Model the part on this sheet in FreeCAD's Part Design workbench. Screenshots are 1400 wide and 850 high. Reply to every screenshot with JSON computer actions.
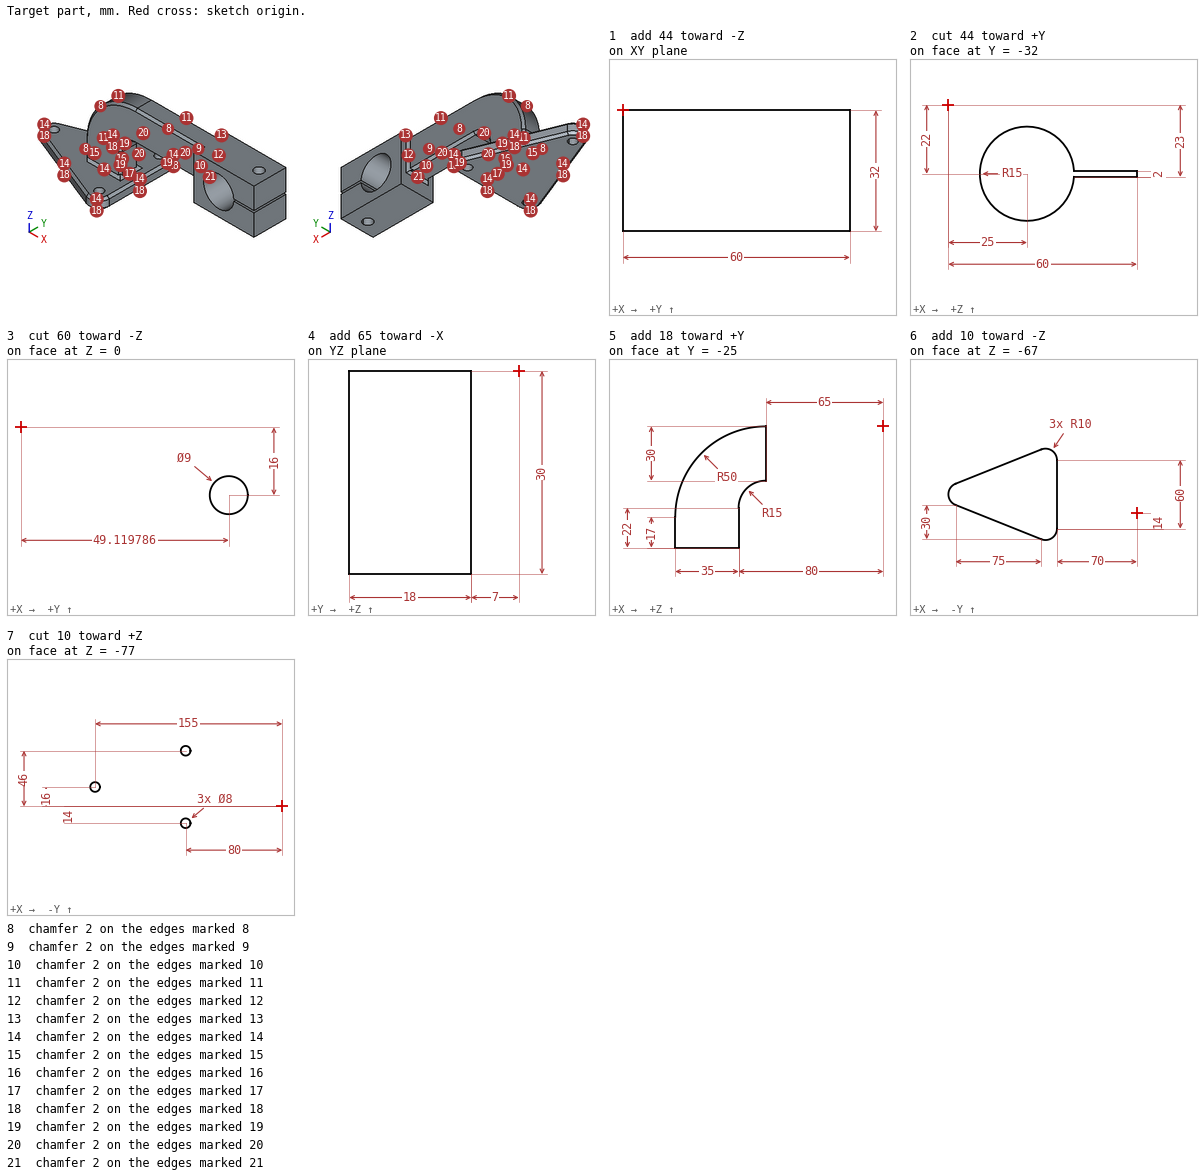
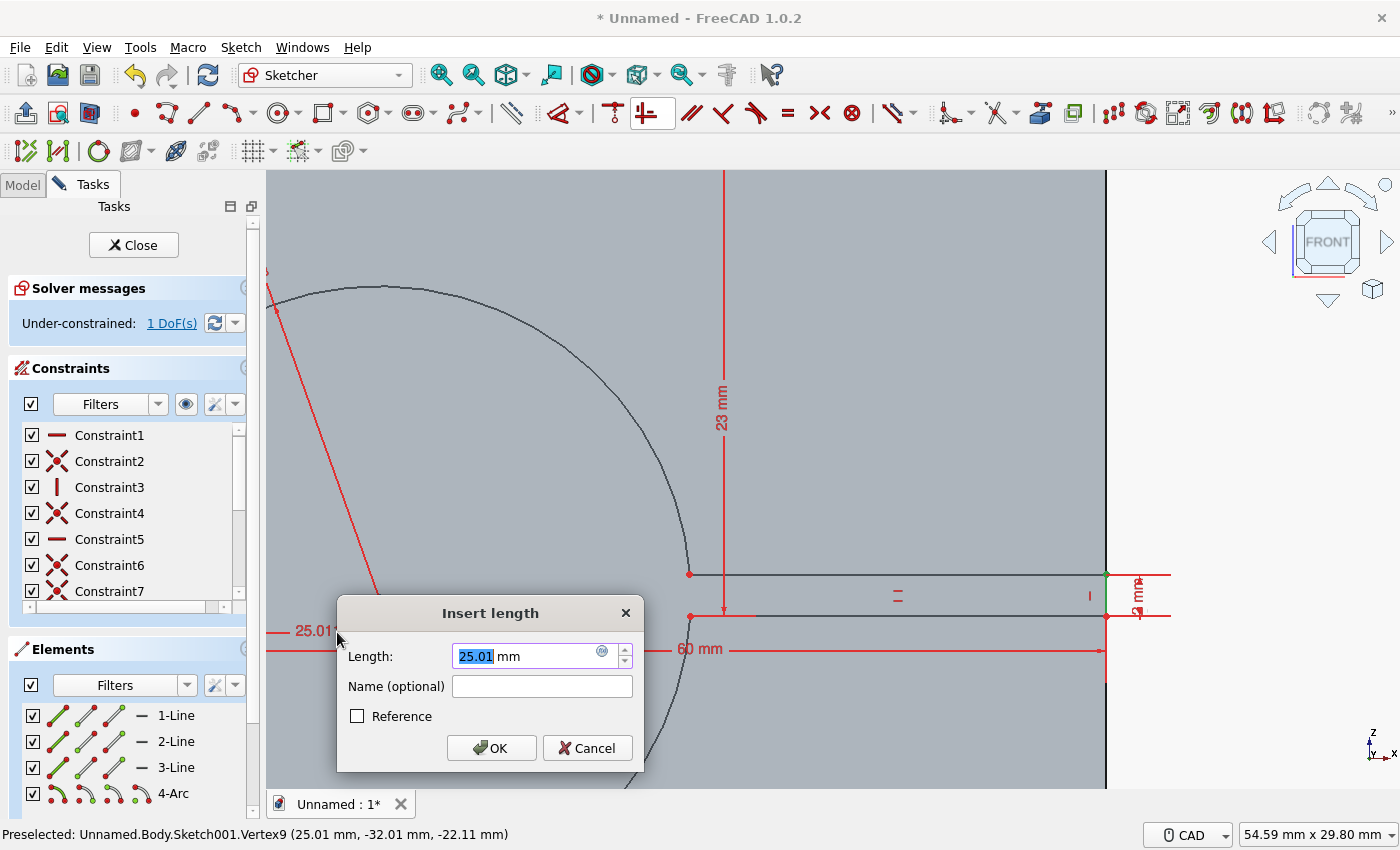
{"action": "type", "text": "25"}
{"action": "key", "text": "Return"}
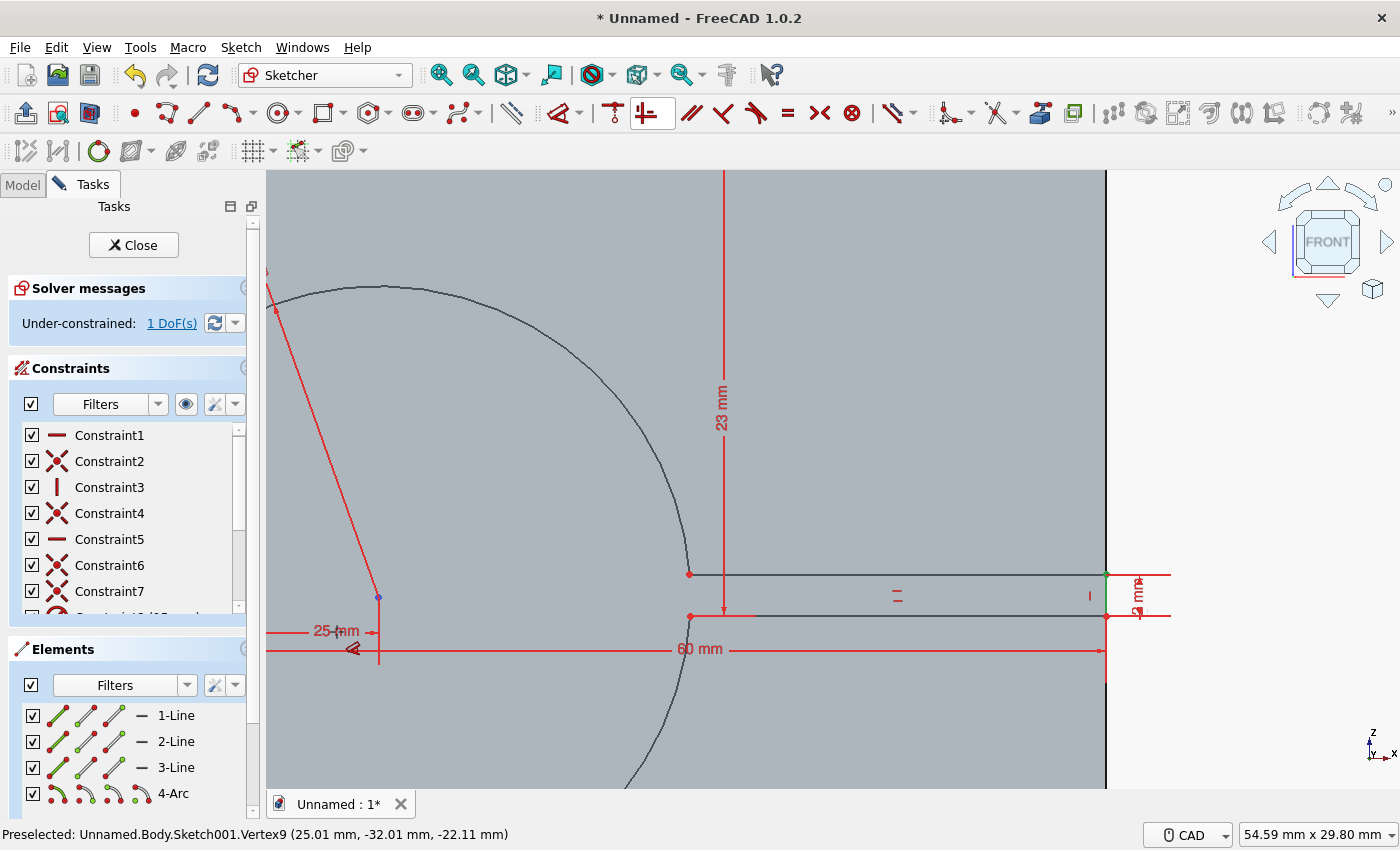
{"action": "left_click", "coordinate": [379, 598]}
{"action": "left_click", "coordinate": [413, 398]}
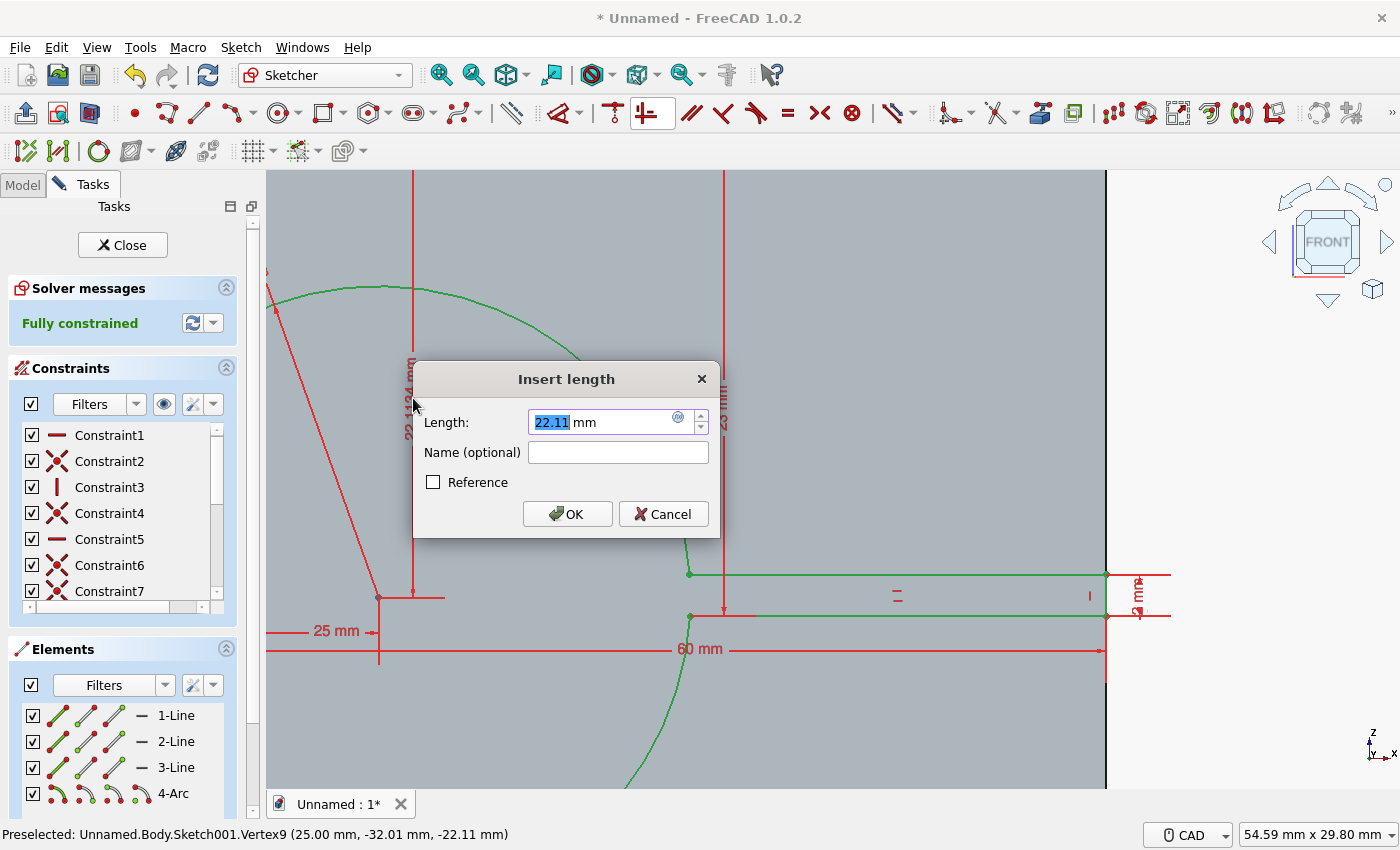
{"action": "type", "text": "22"}
{"action": "key", "text": "Return"}
{"action": "key", "text": "Escape"}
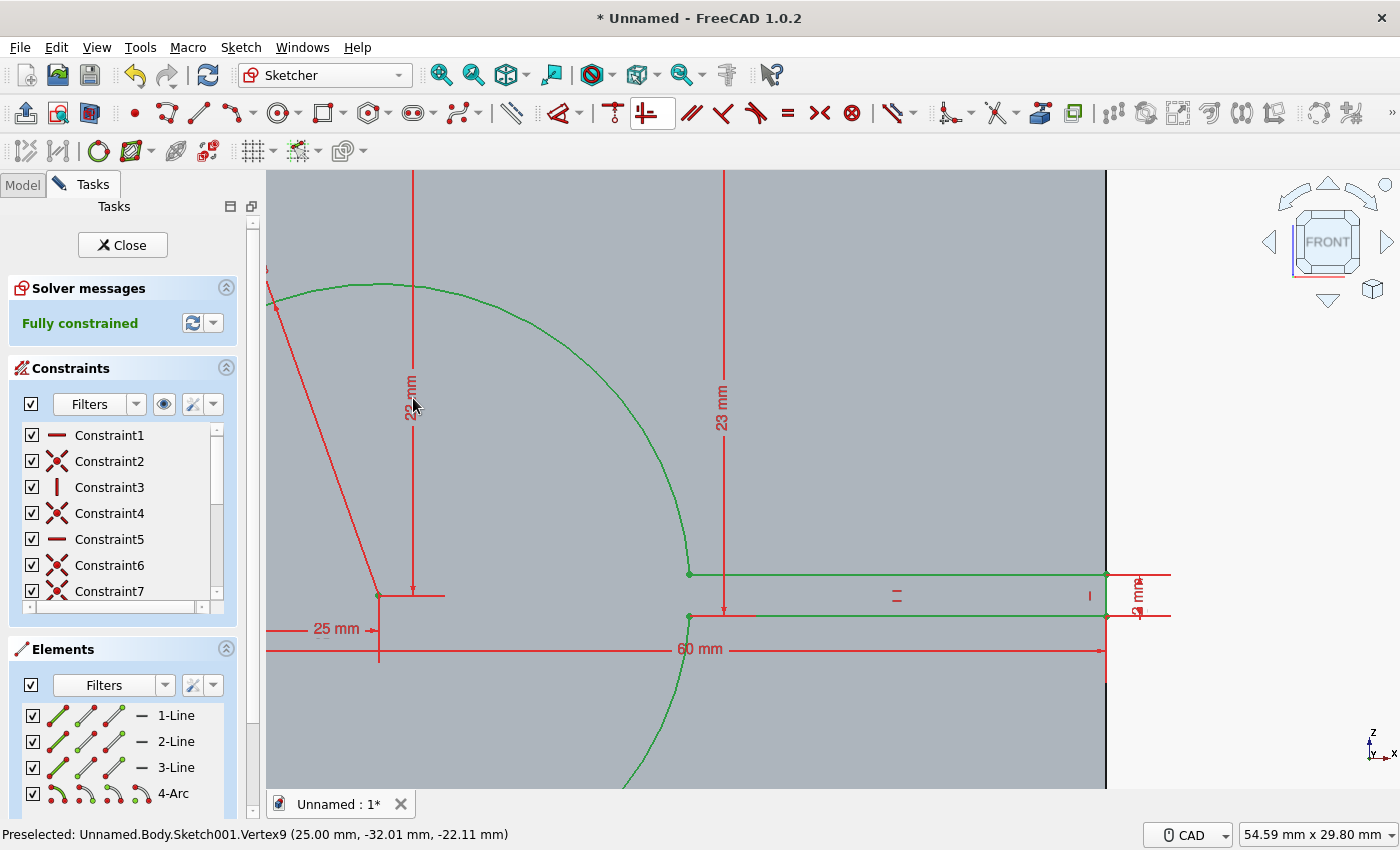
{"action": "left_click", "coordinate": [123, 245]}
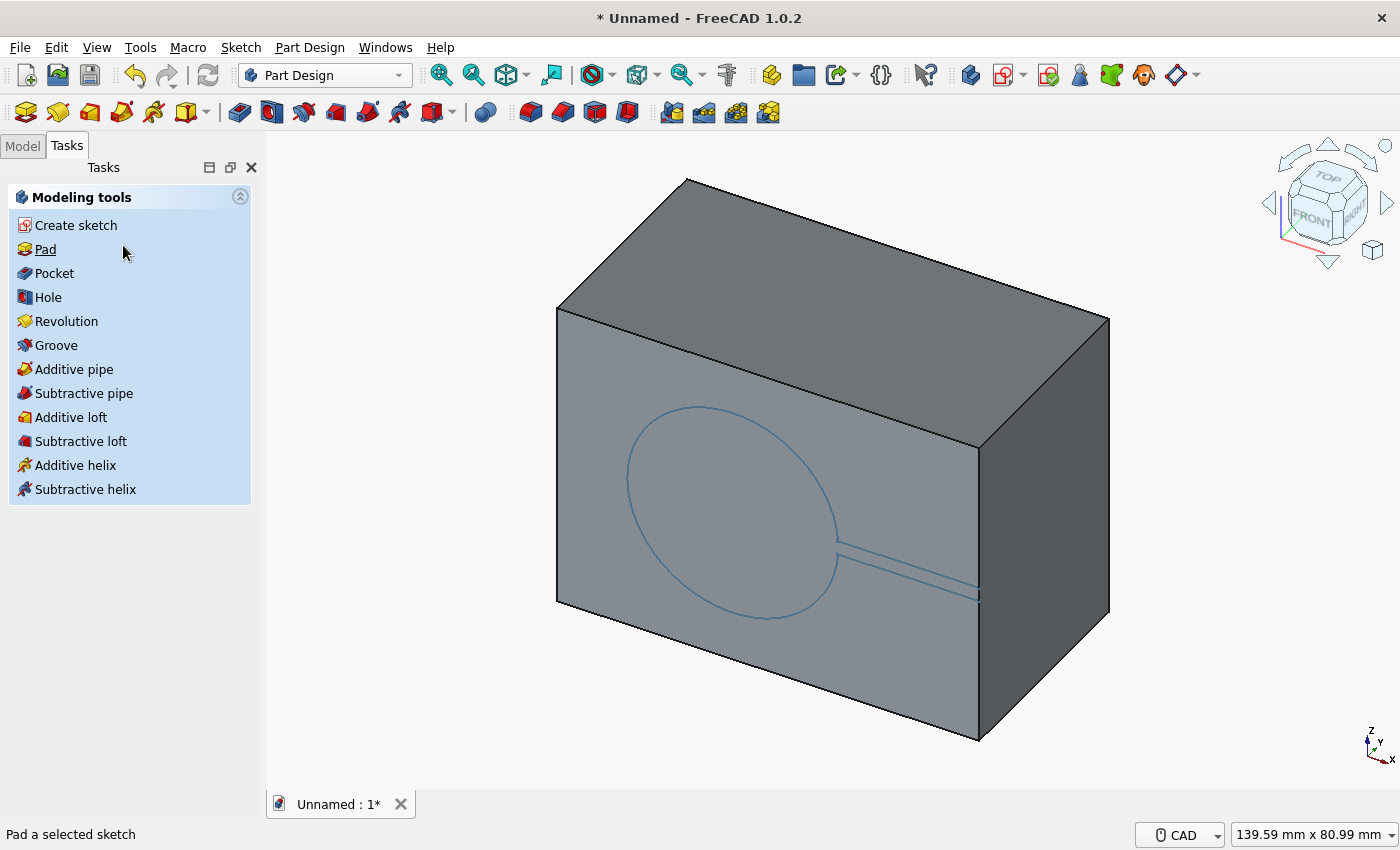
{"action": "left_click", "coordinate": [240, 112]}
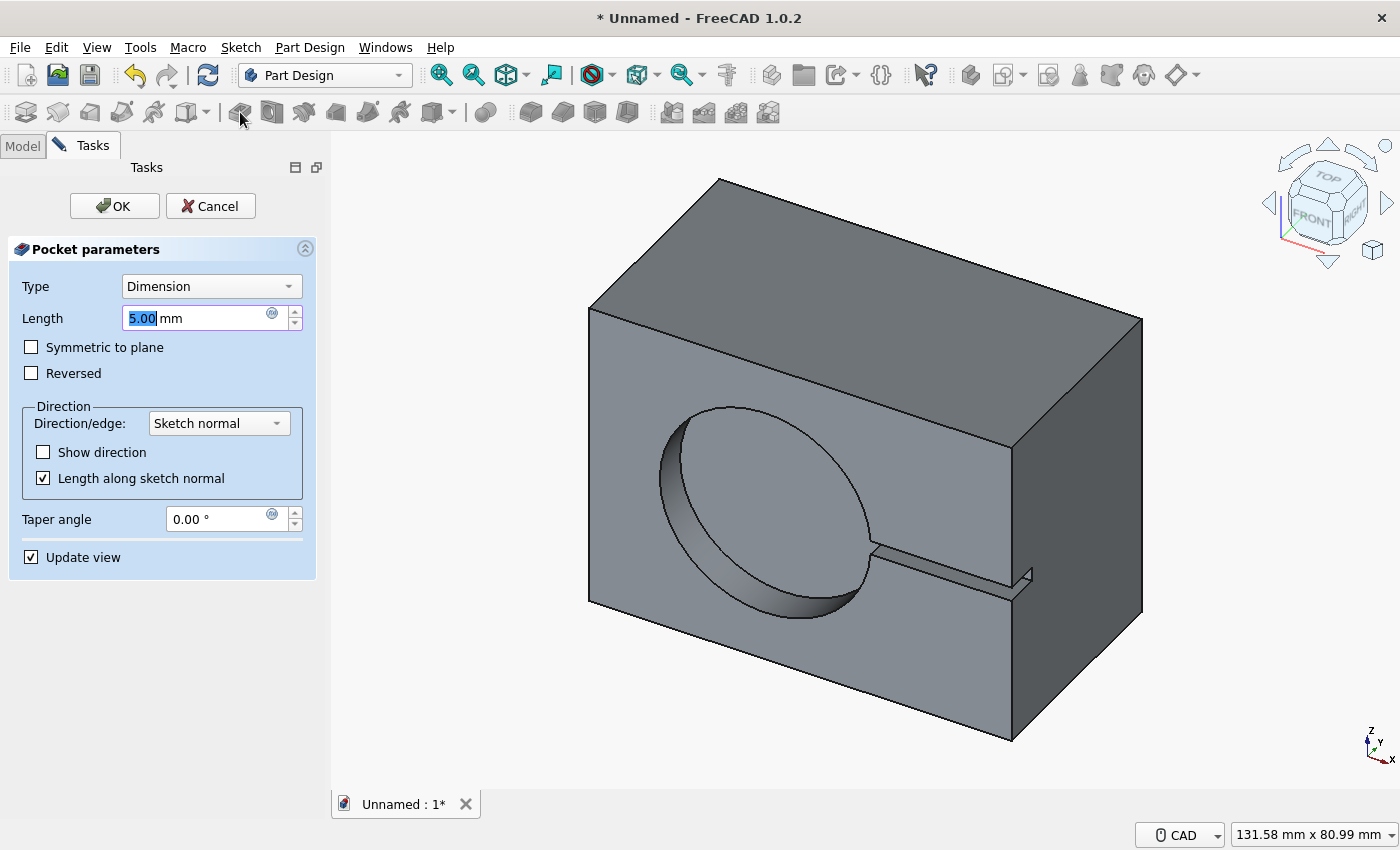
{"action": "type", "text": "44"}
{"action": "key", "text": "Tab"}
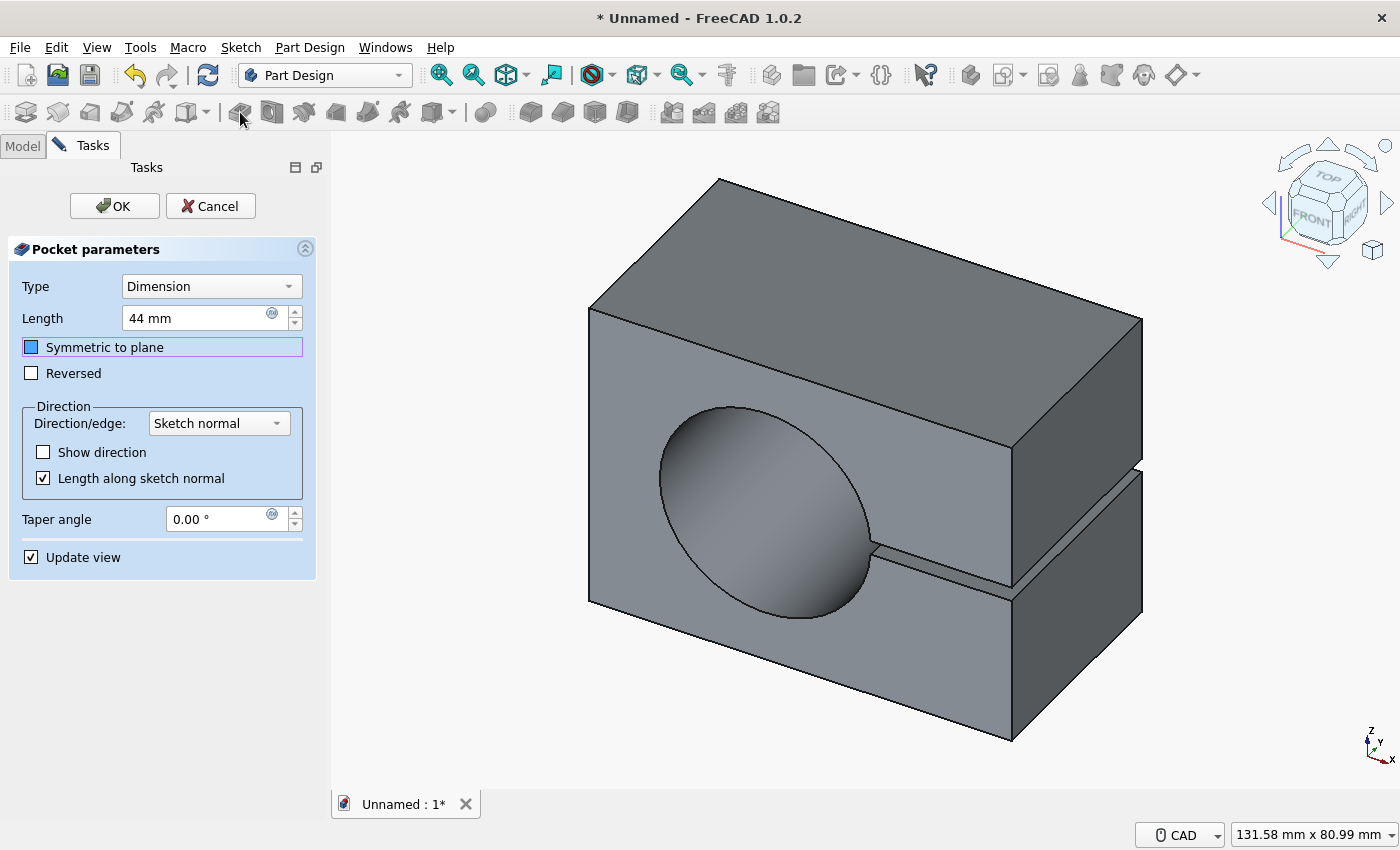
{"action": "left_click", "coordinate": [115, 206]}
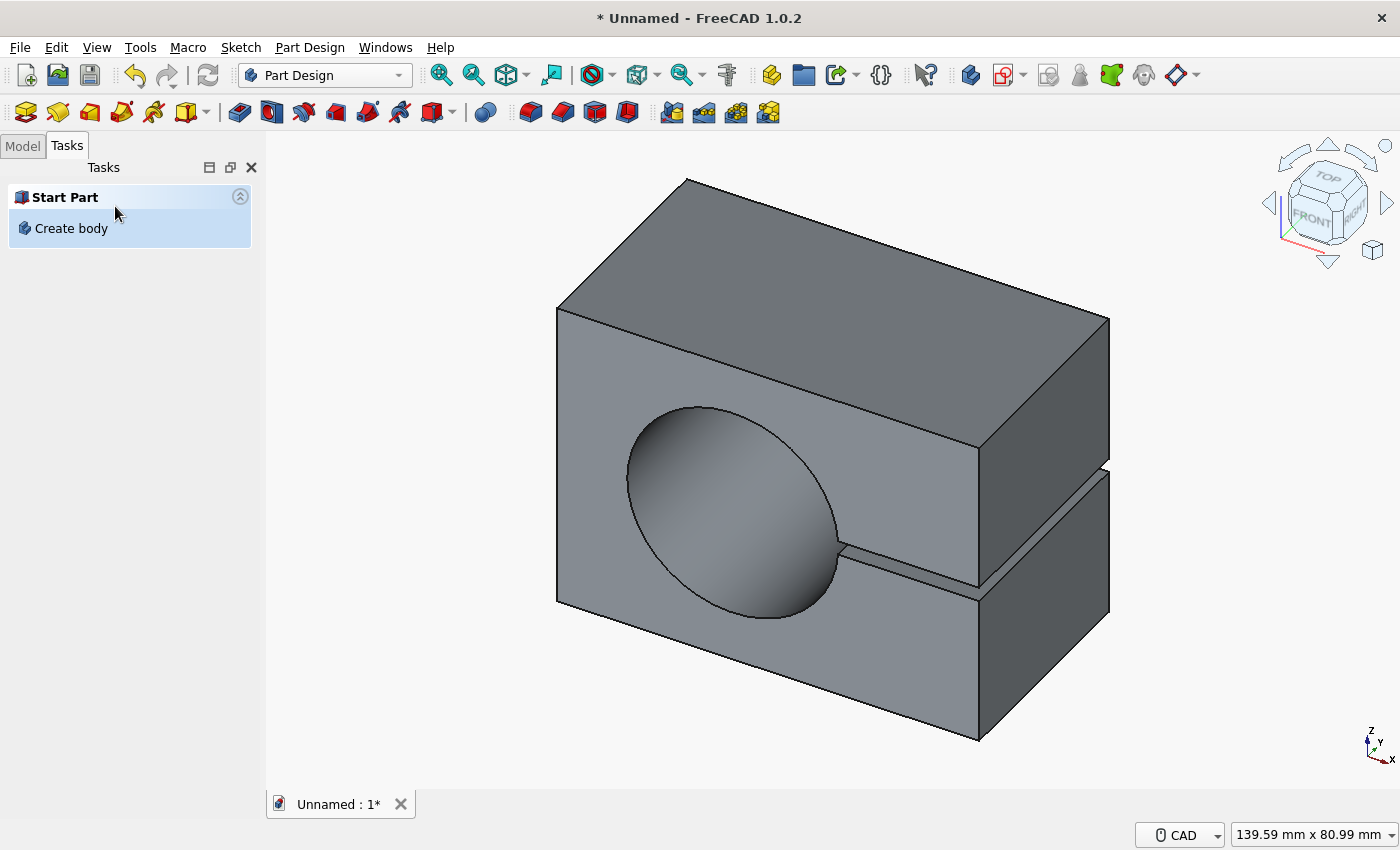
{"action": "left_click", "coordinate": [893, 333]}